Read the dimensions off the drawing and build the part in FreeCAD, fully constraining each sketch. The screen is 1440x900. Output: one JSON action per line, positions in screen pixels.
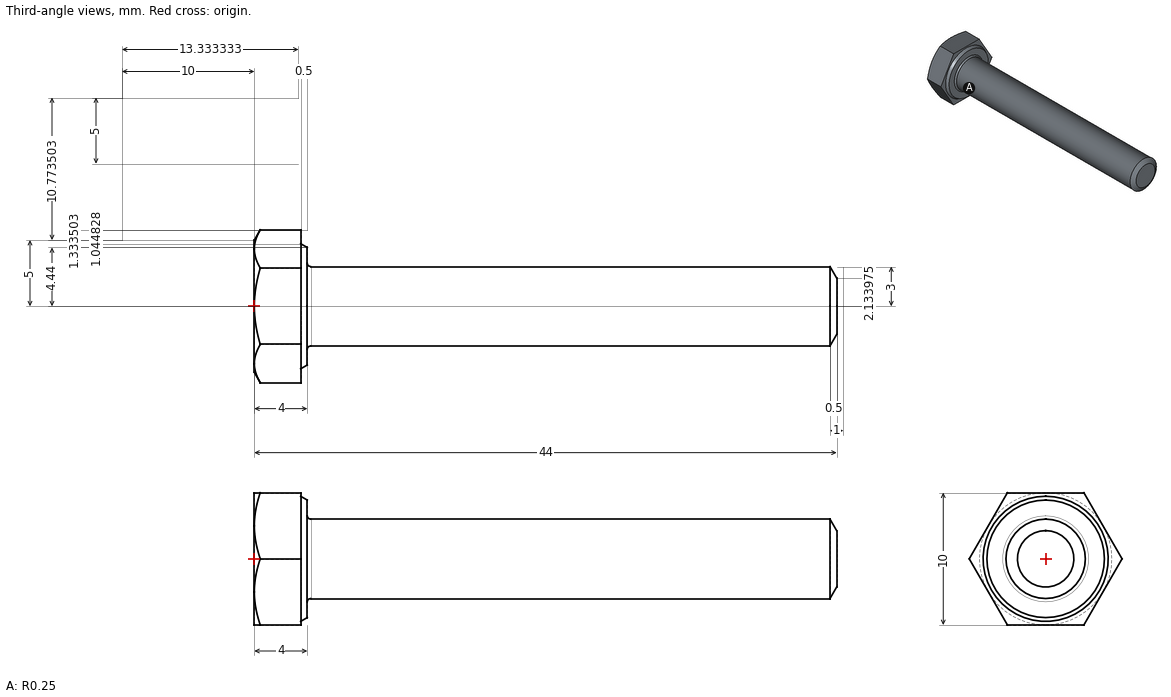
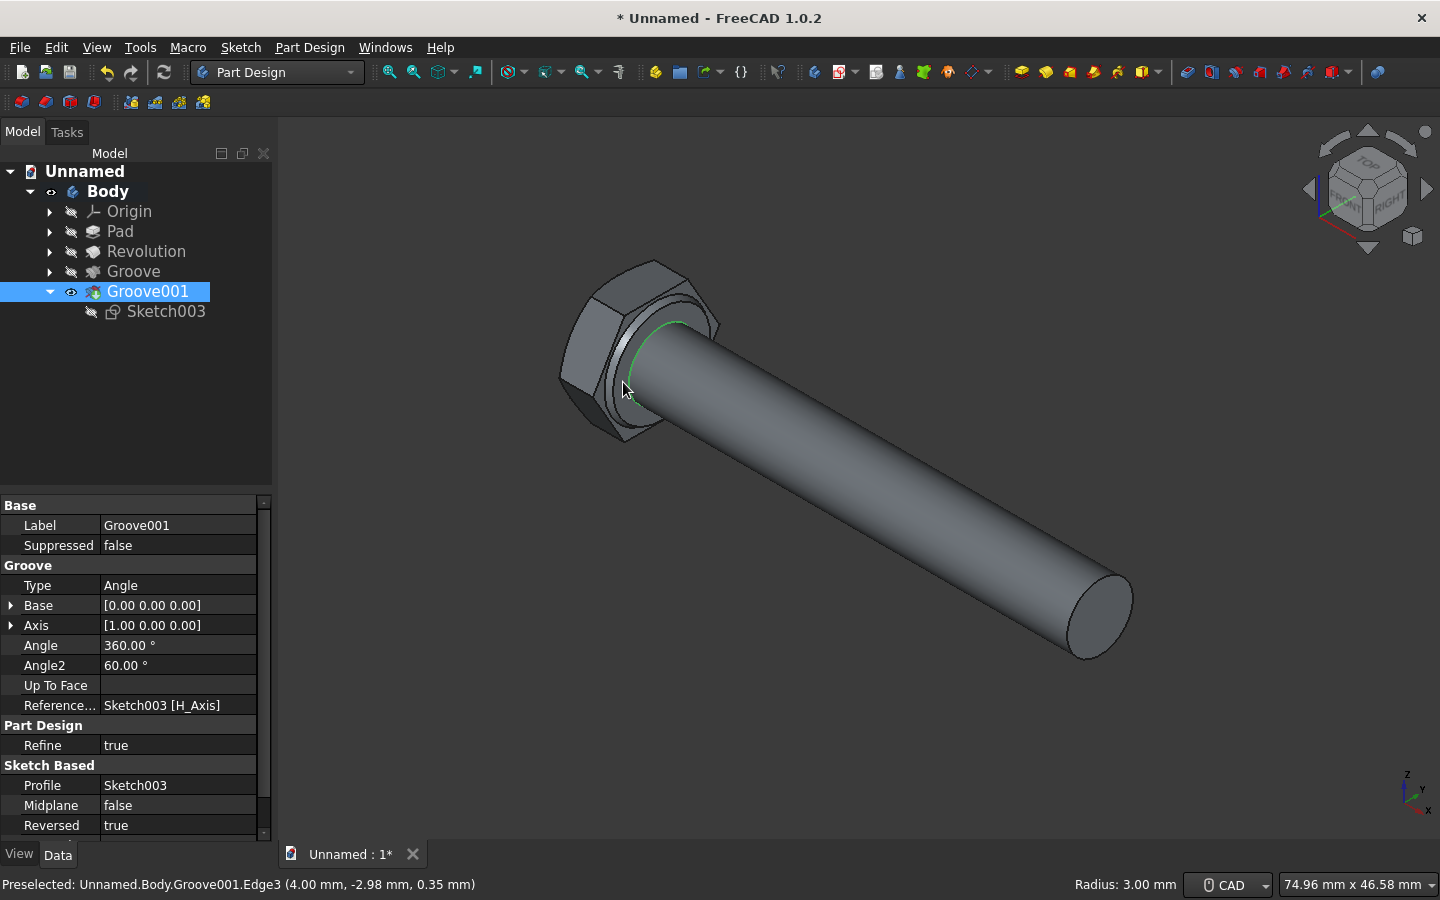
{"action": "left_click", "coordinate": [22, 102]}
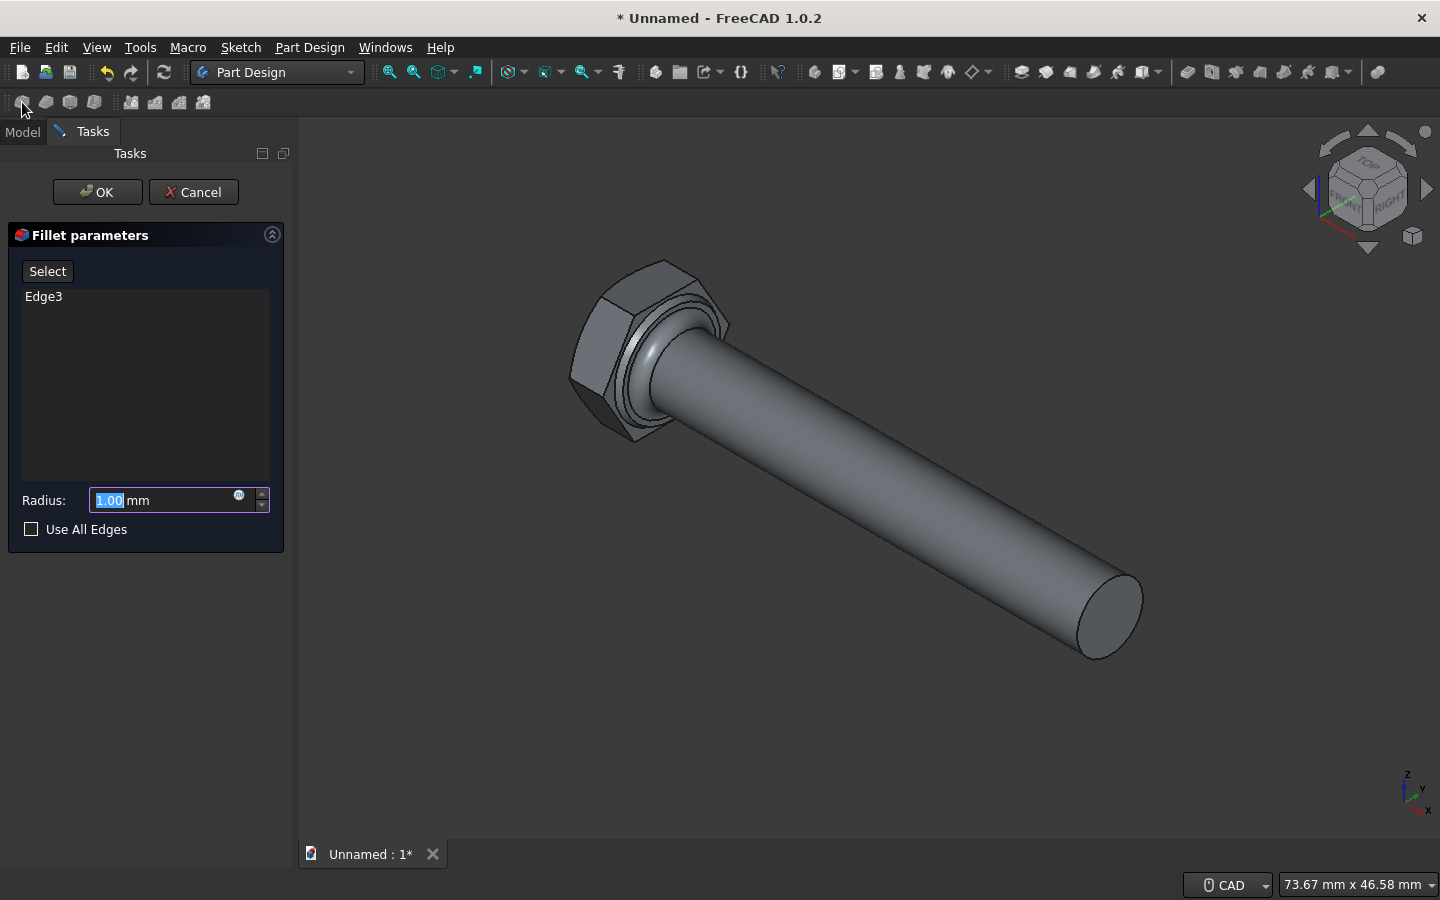
{"action": "type", "text": "0.25"}
{"action": "key", "text": "Tab"}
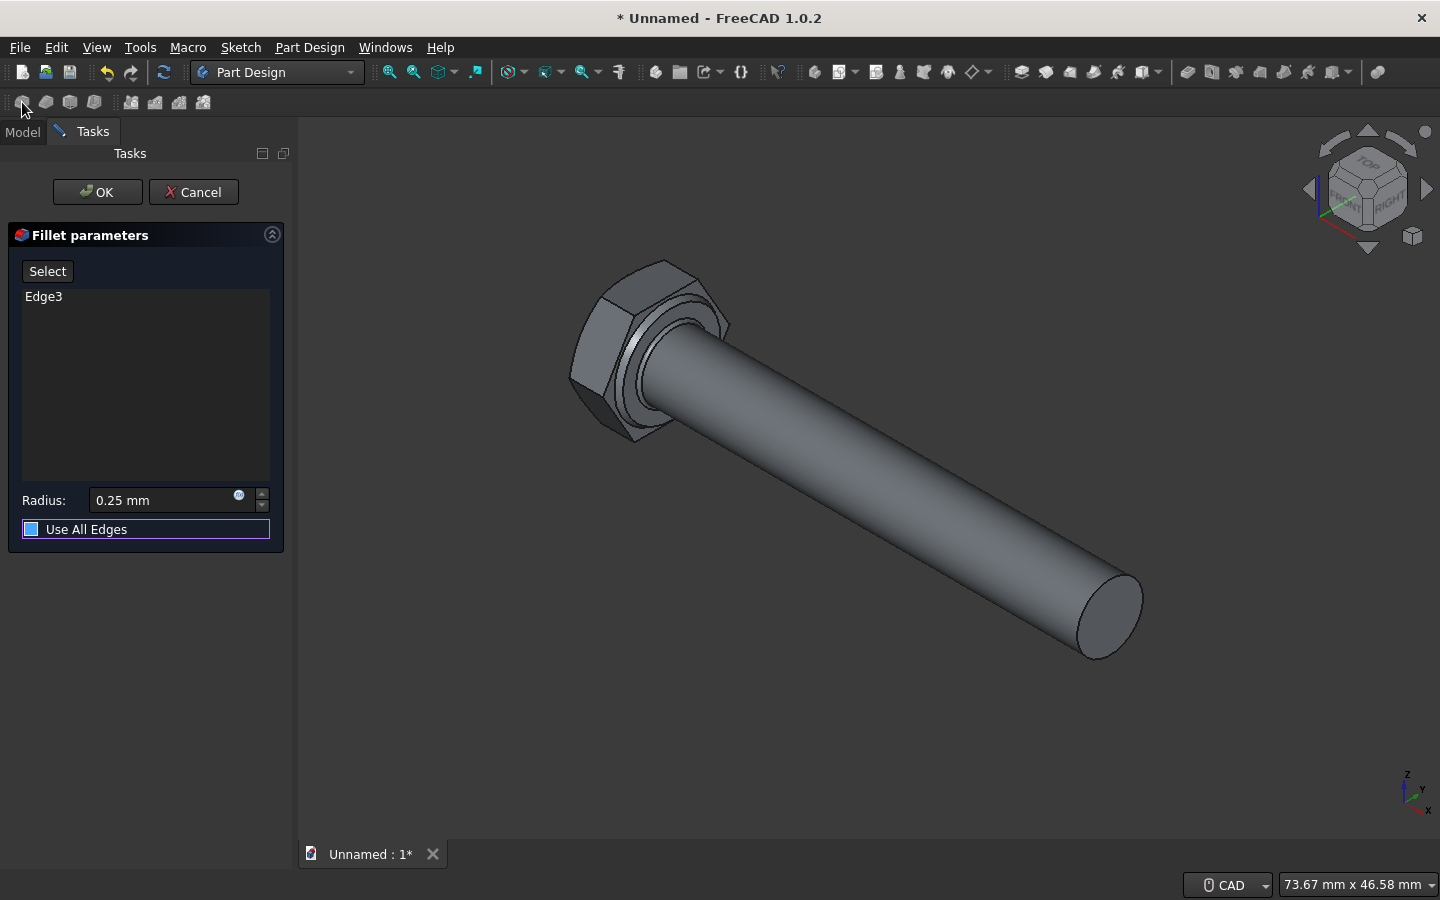
{"action": "left_click", "coordinate": [98, 192]}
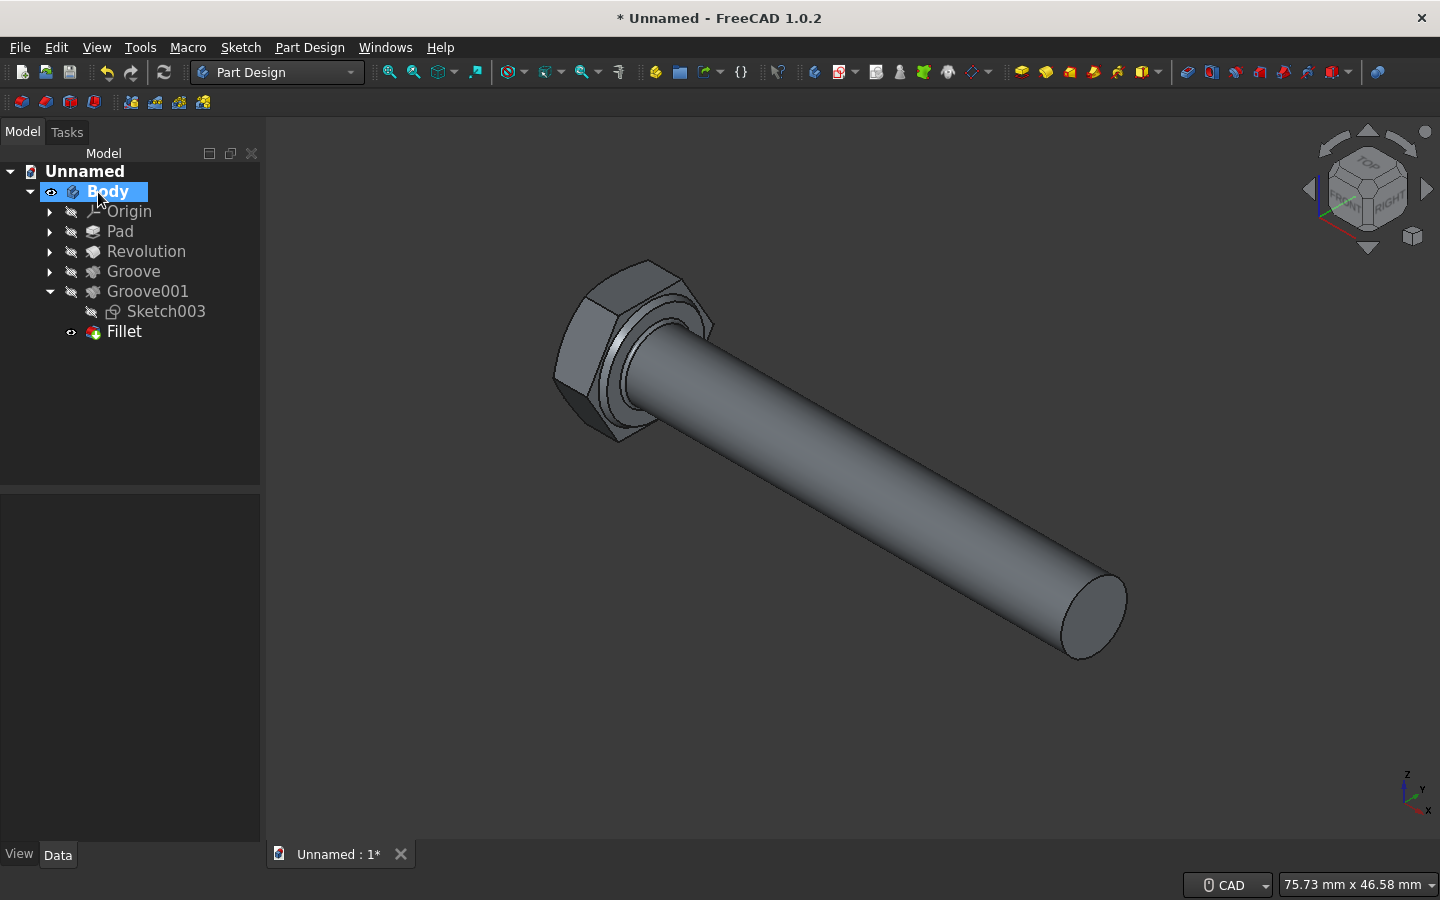
{"action": "left_click", "coordinate": [840, 72]}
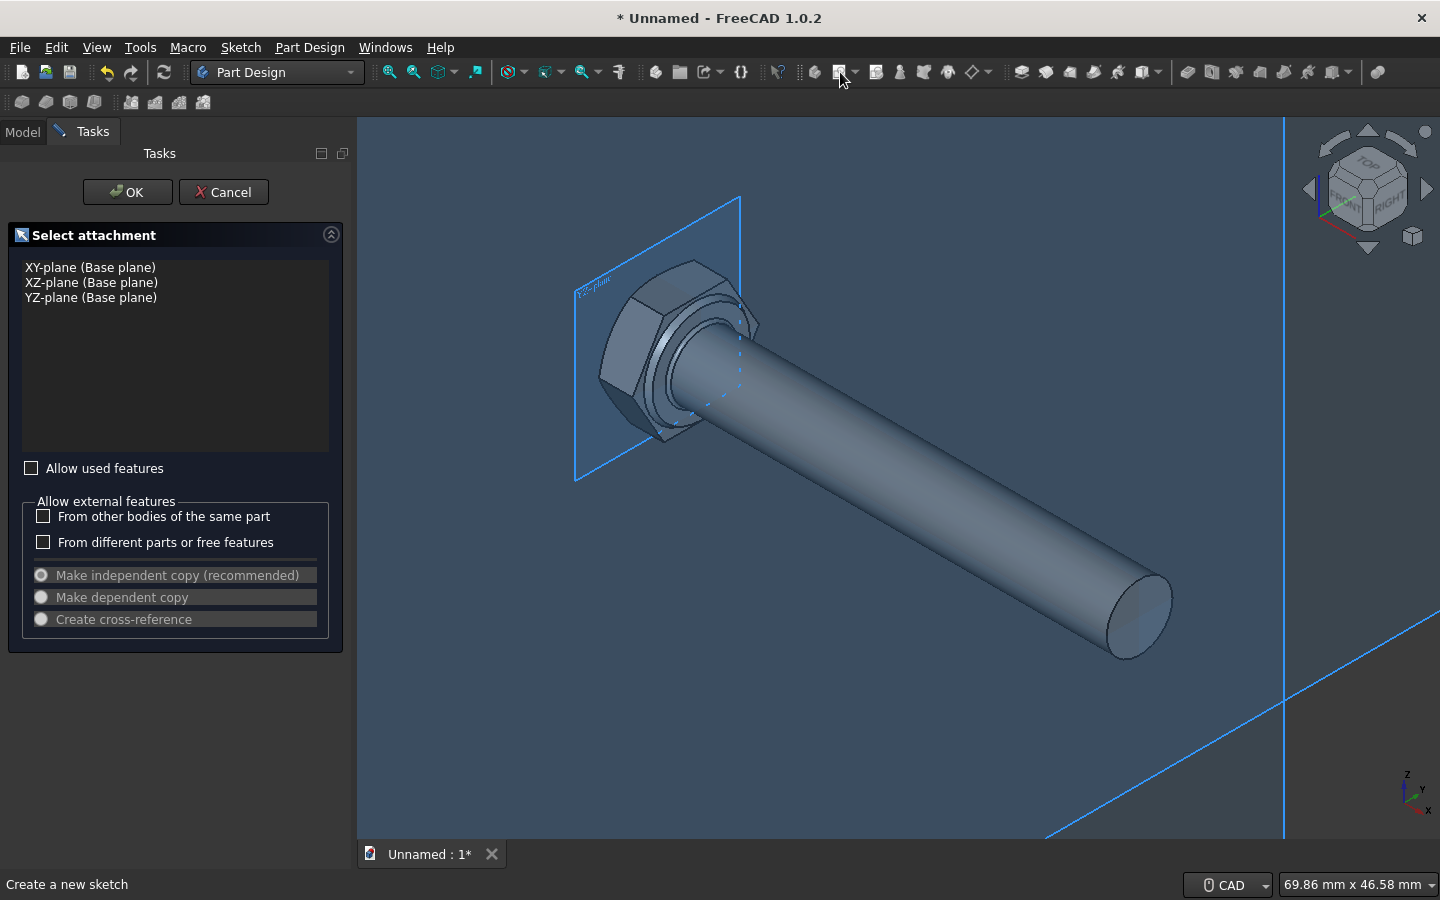
{"action": "left_click", "coordinate": [82, 268]}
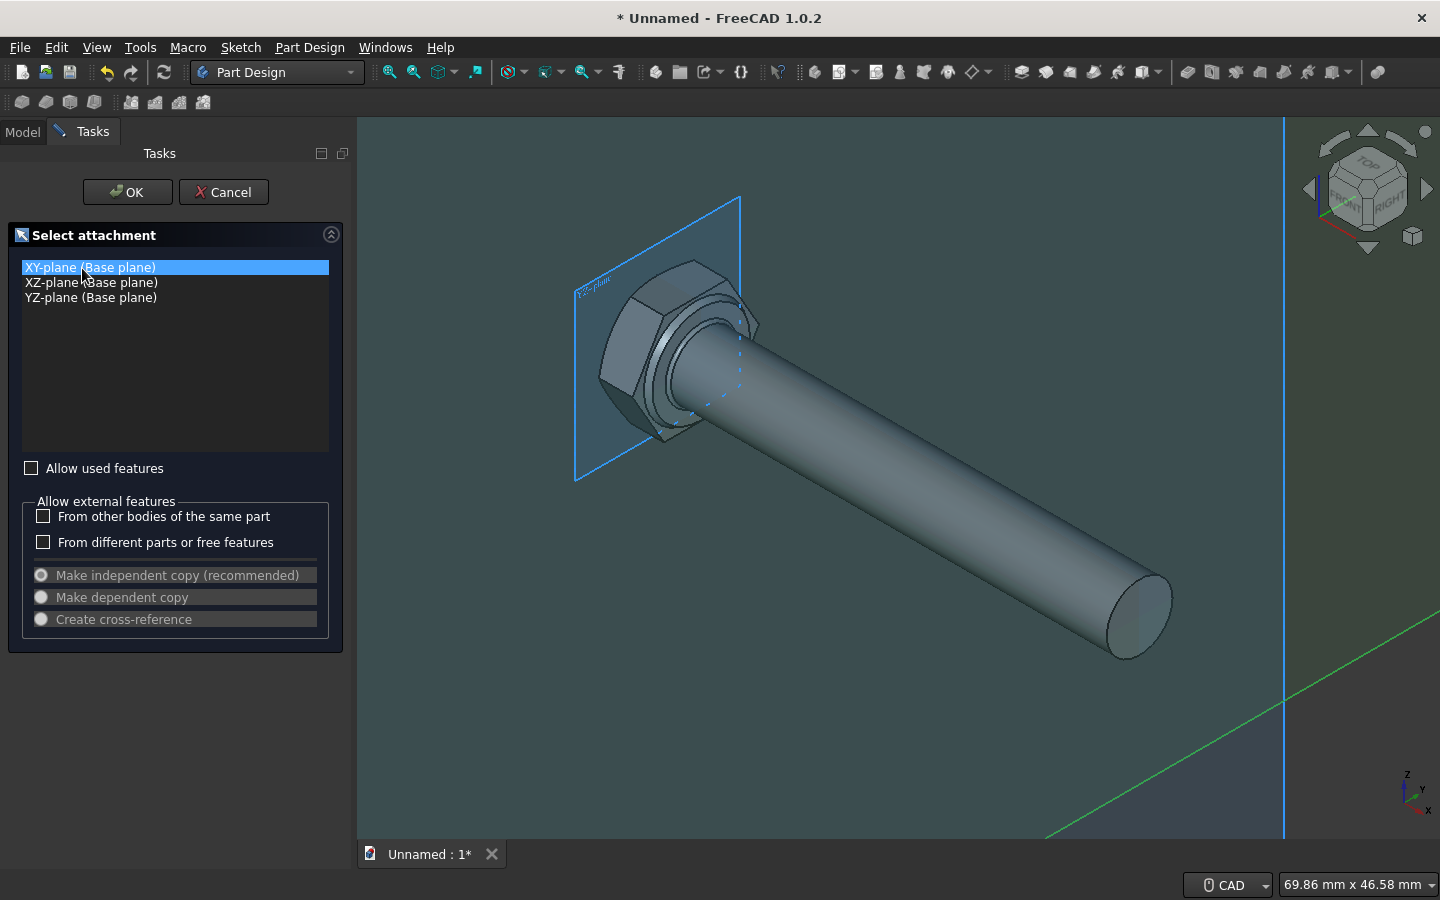
{"action": "left_click", "coordinate": [128, 192]}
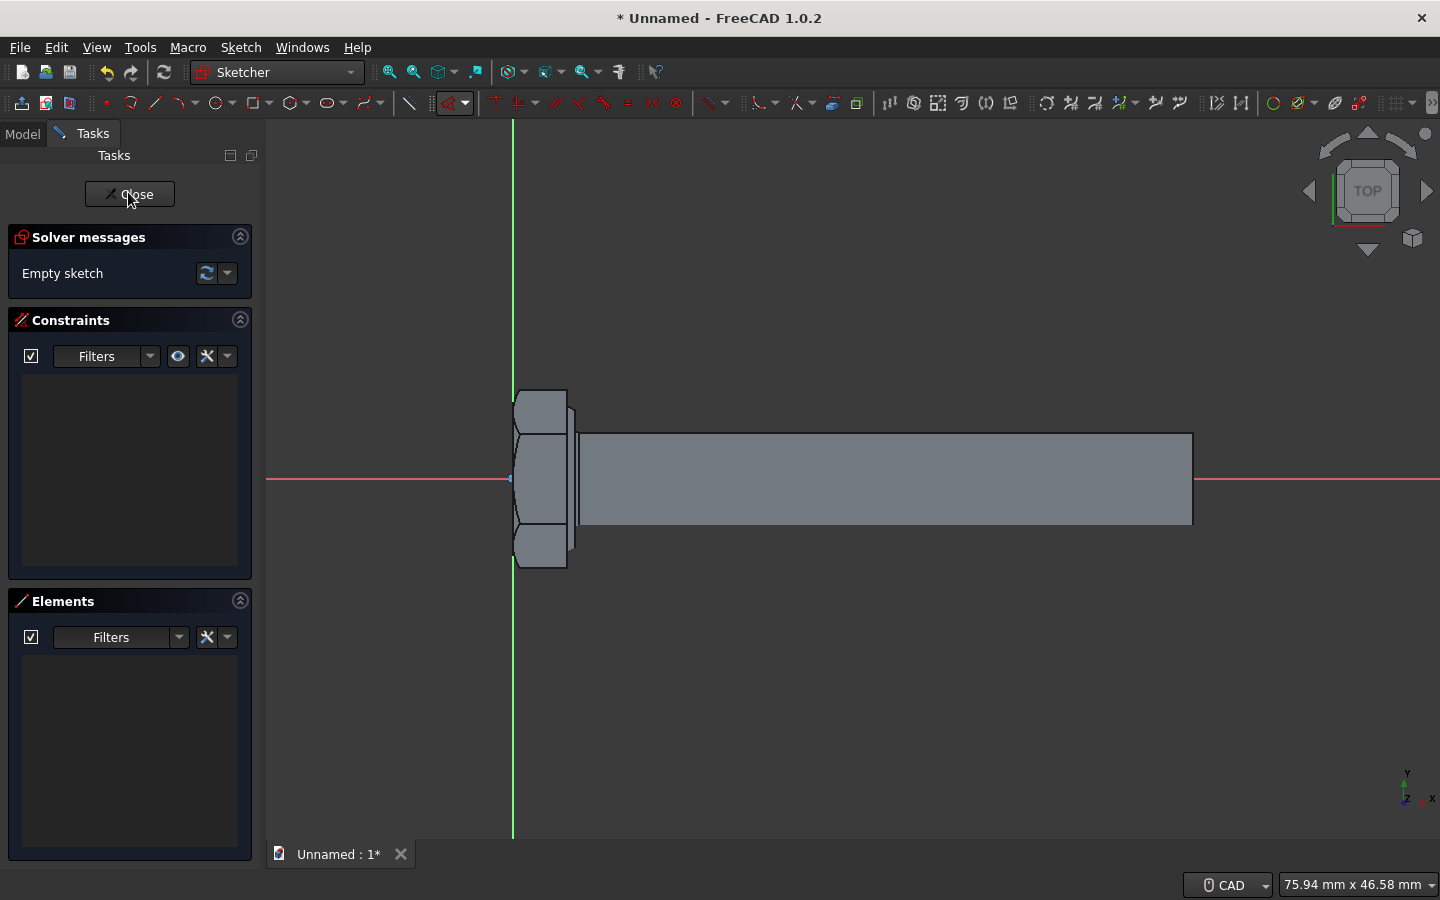
{"action": "left_click", "coordinate": [70, 104]}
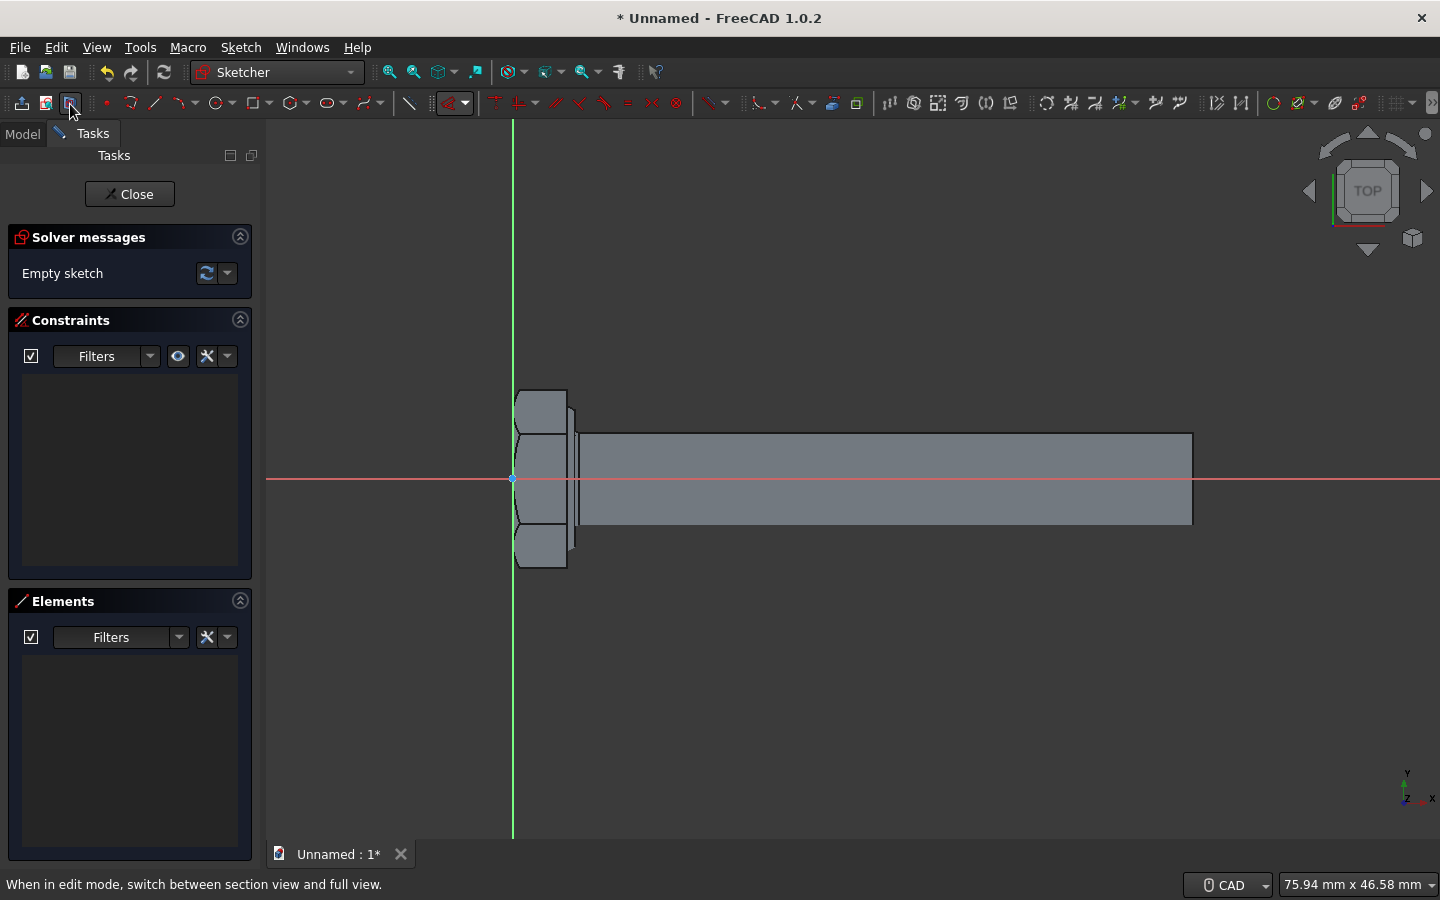
{"action": "scroll", "coordinate": [1214, 437], "scroll_direction": "up", "scroll_amount": 15}